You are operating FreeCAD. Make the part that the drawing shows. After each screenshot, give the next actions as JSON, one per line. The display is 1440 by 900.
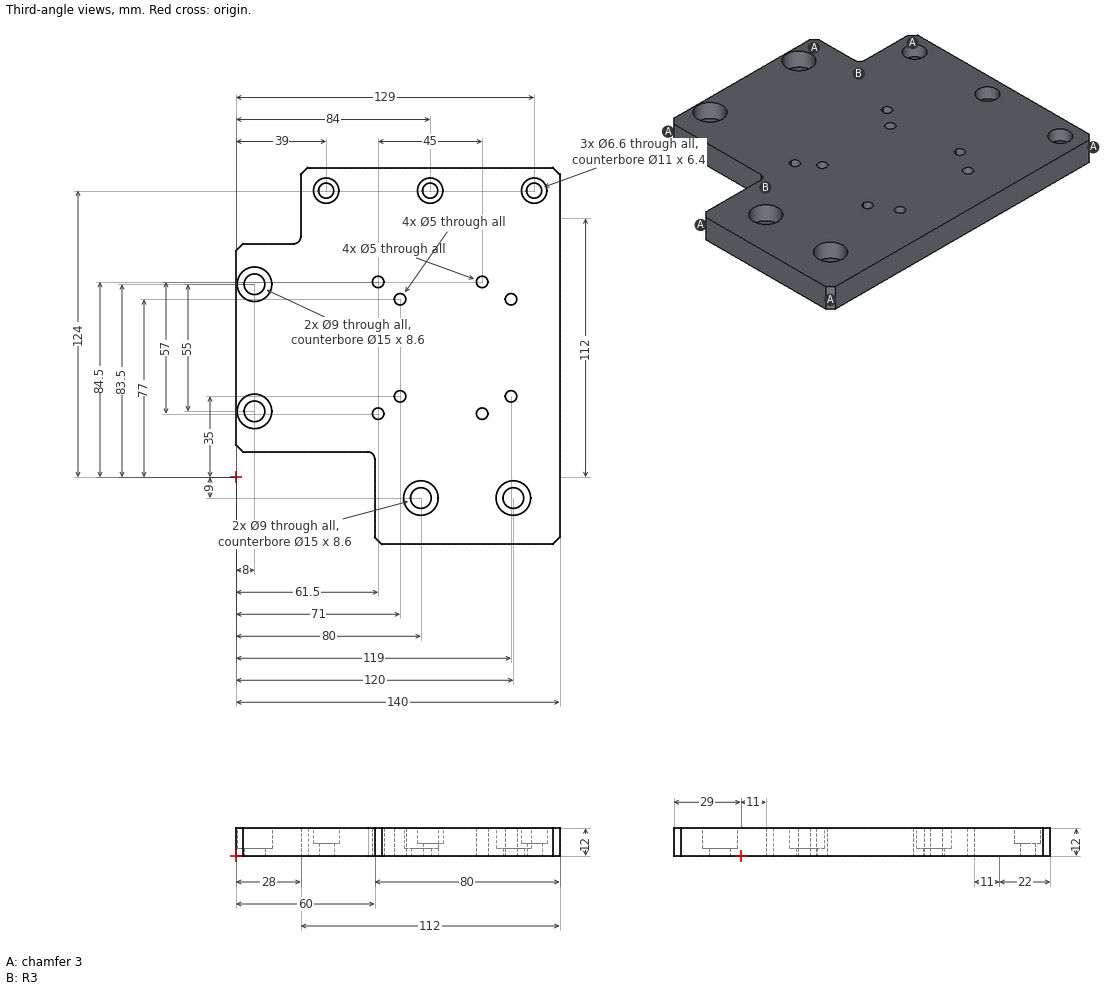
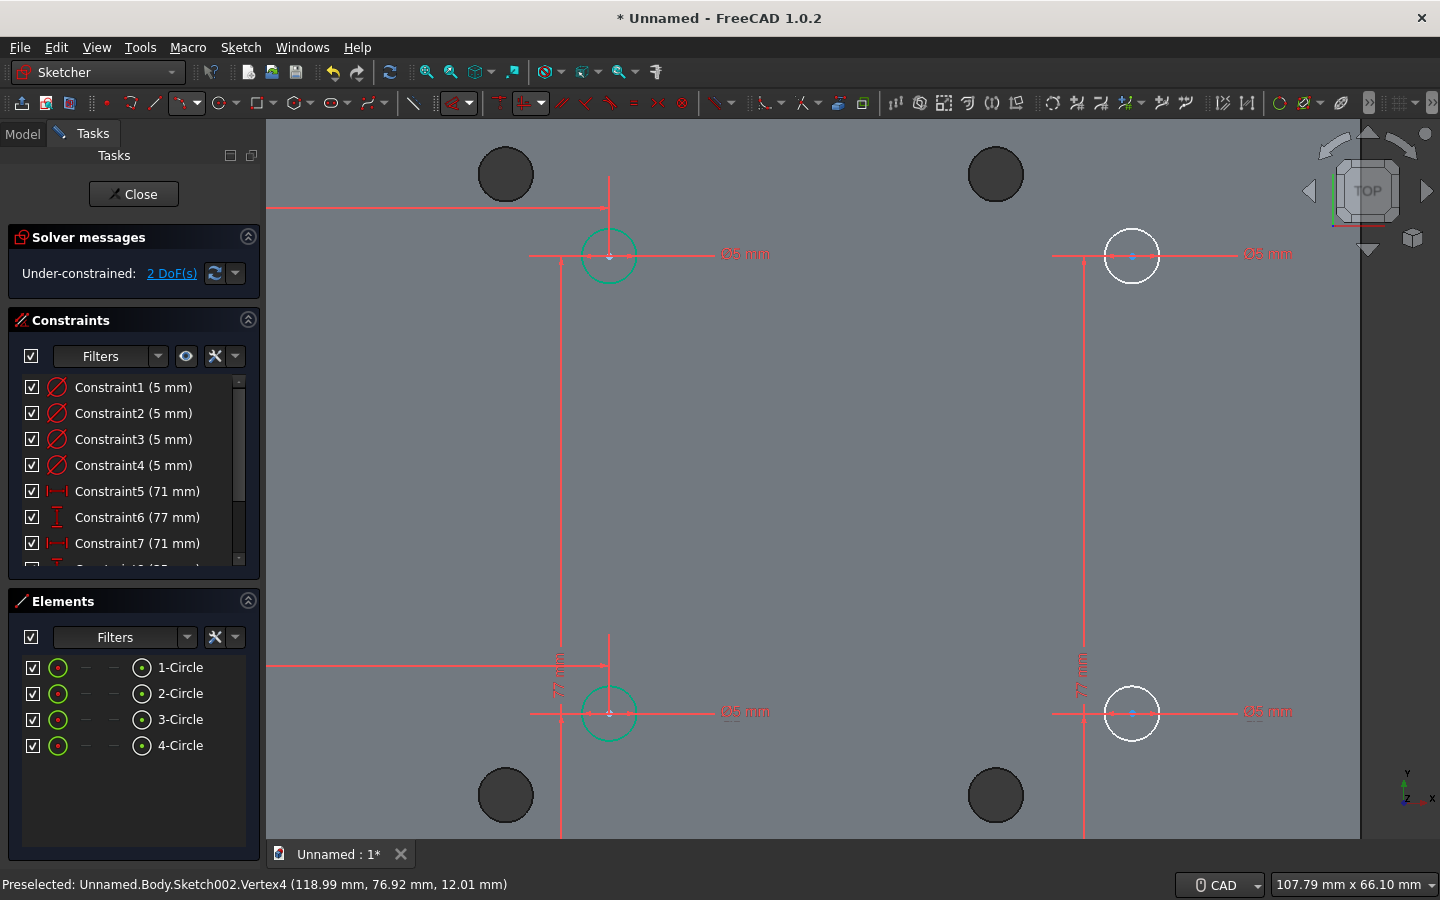
{"action": "left_click", "coordinate": [1132, 714]}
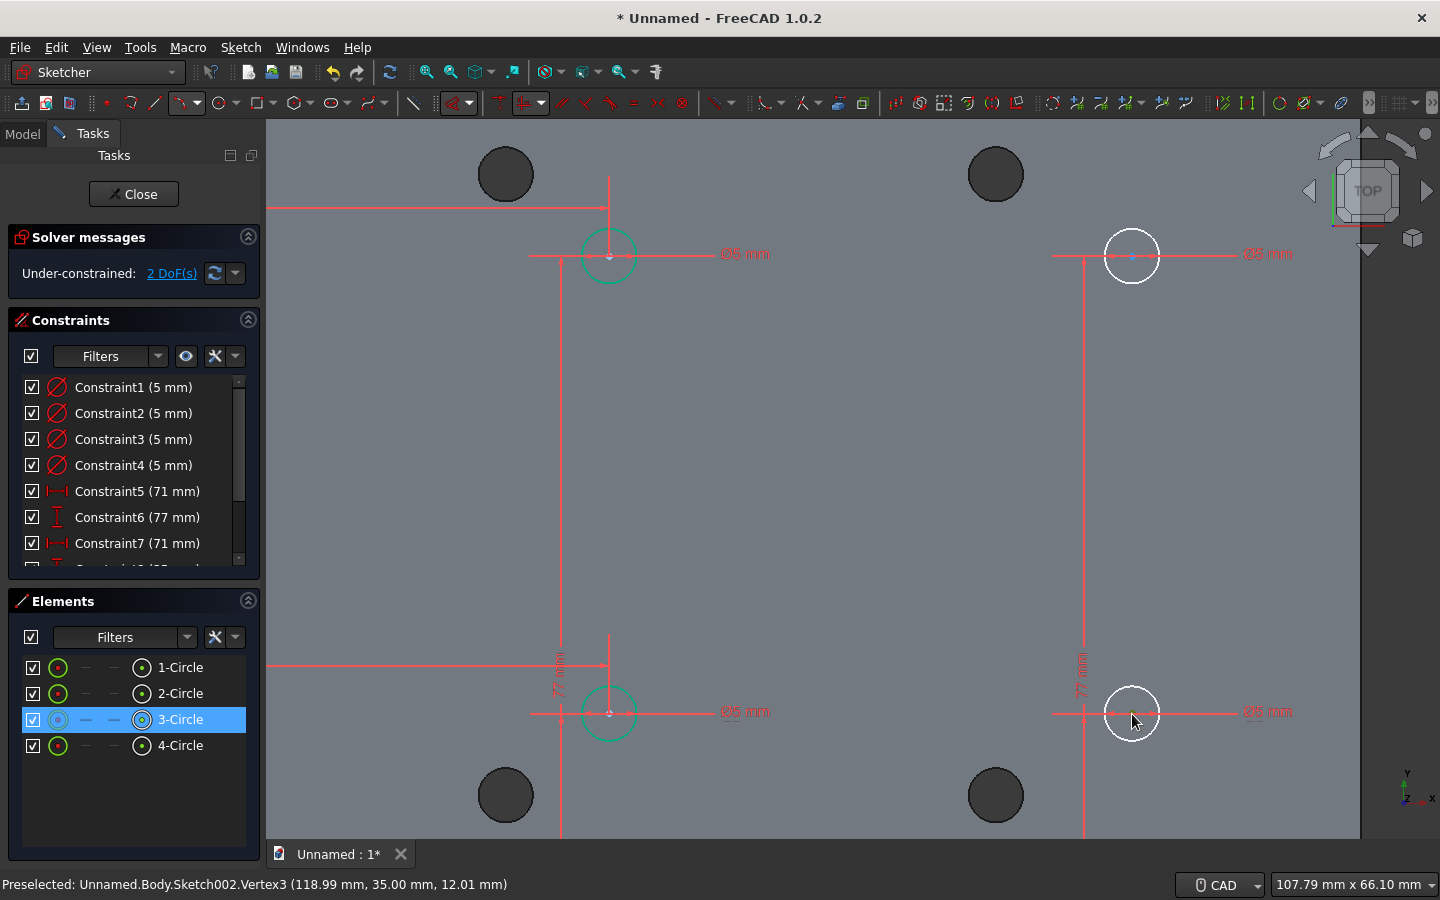
{"action": "key", "text": "l"}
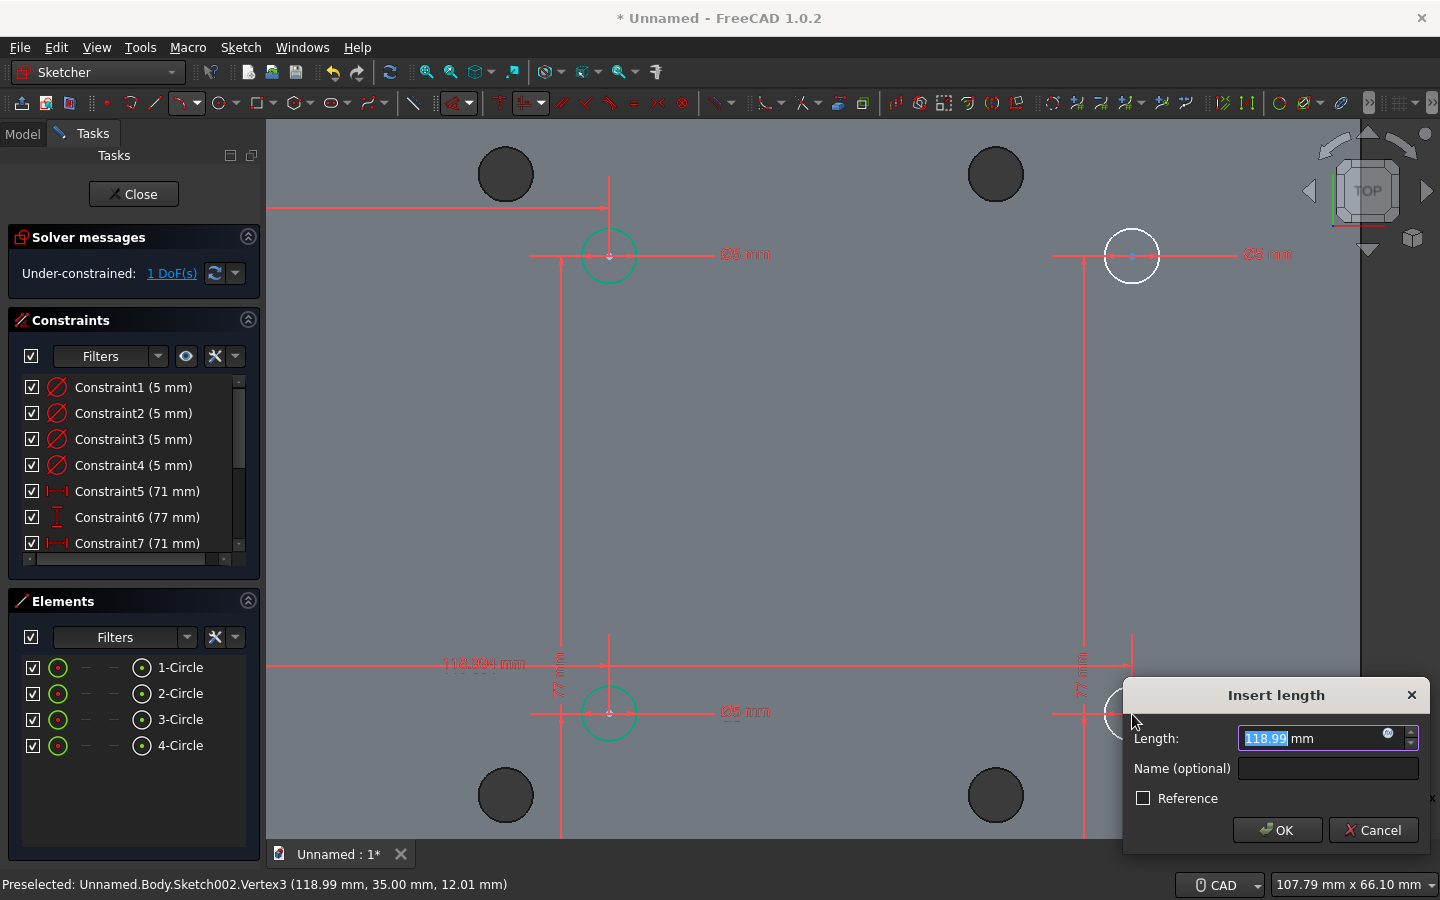
{"action": "type", "text": "119"}
{"action": "key", "text": "Return"}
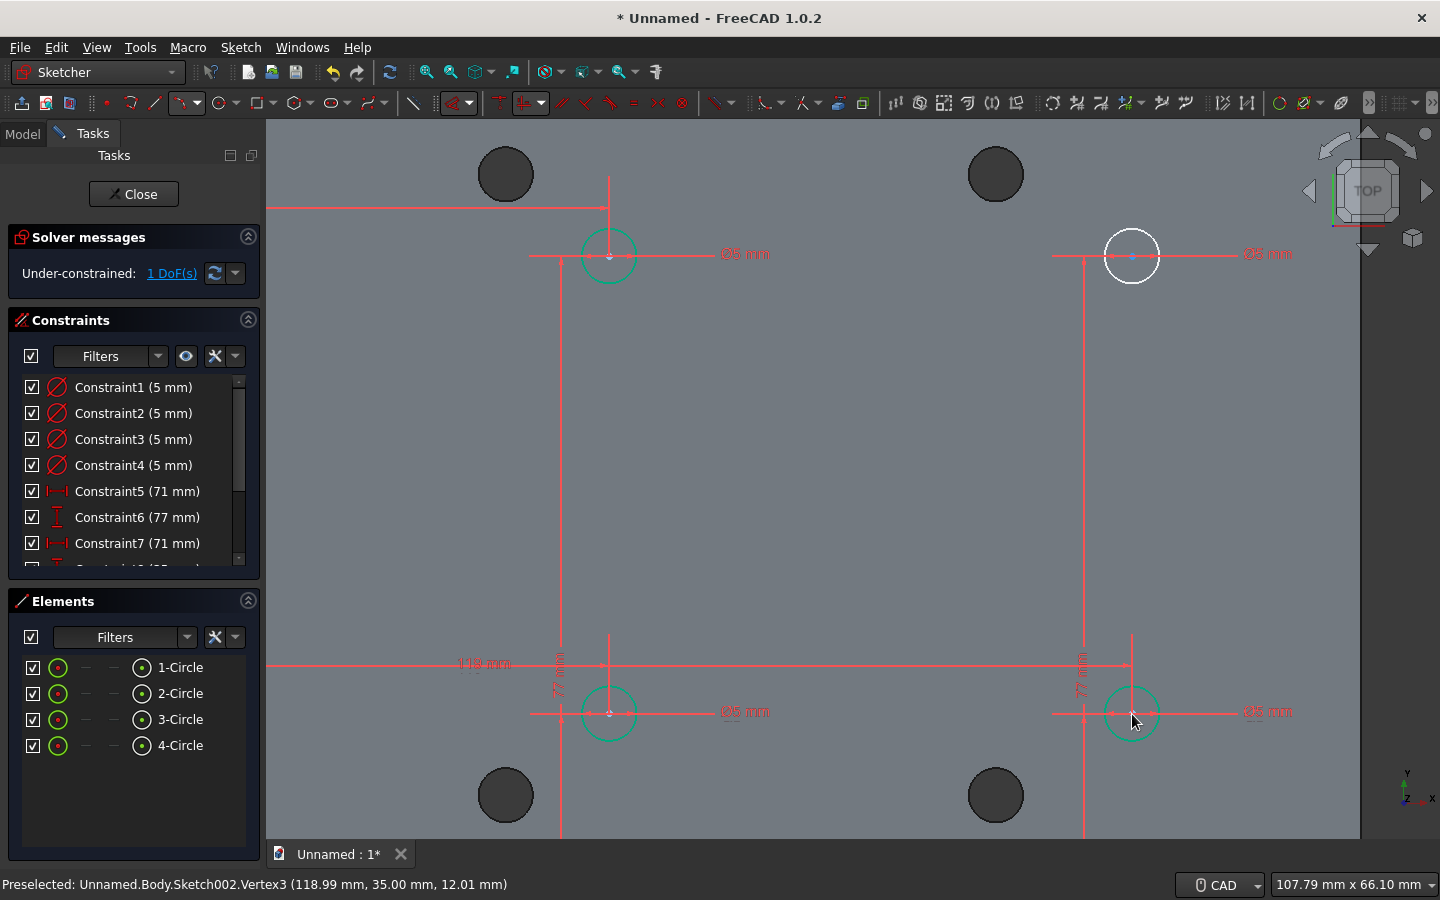
{"action": "left_click", "coordinate": [1132, 256]}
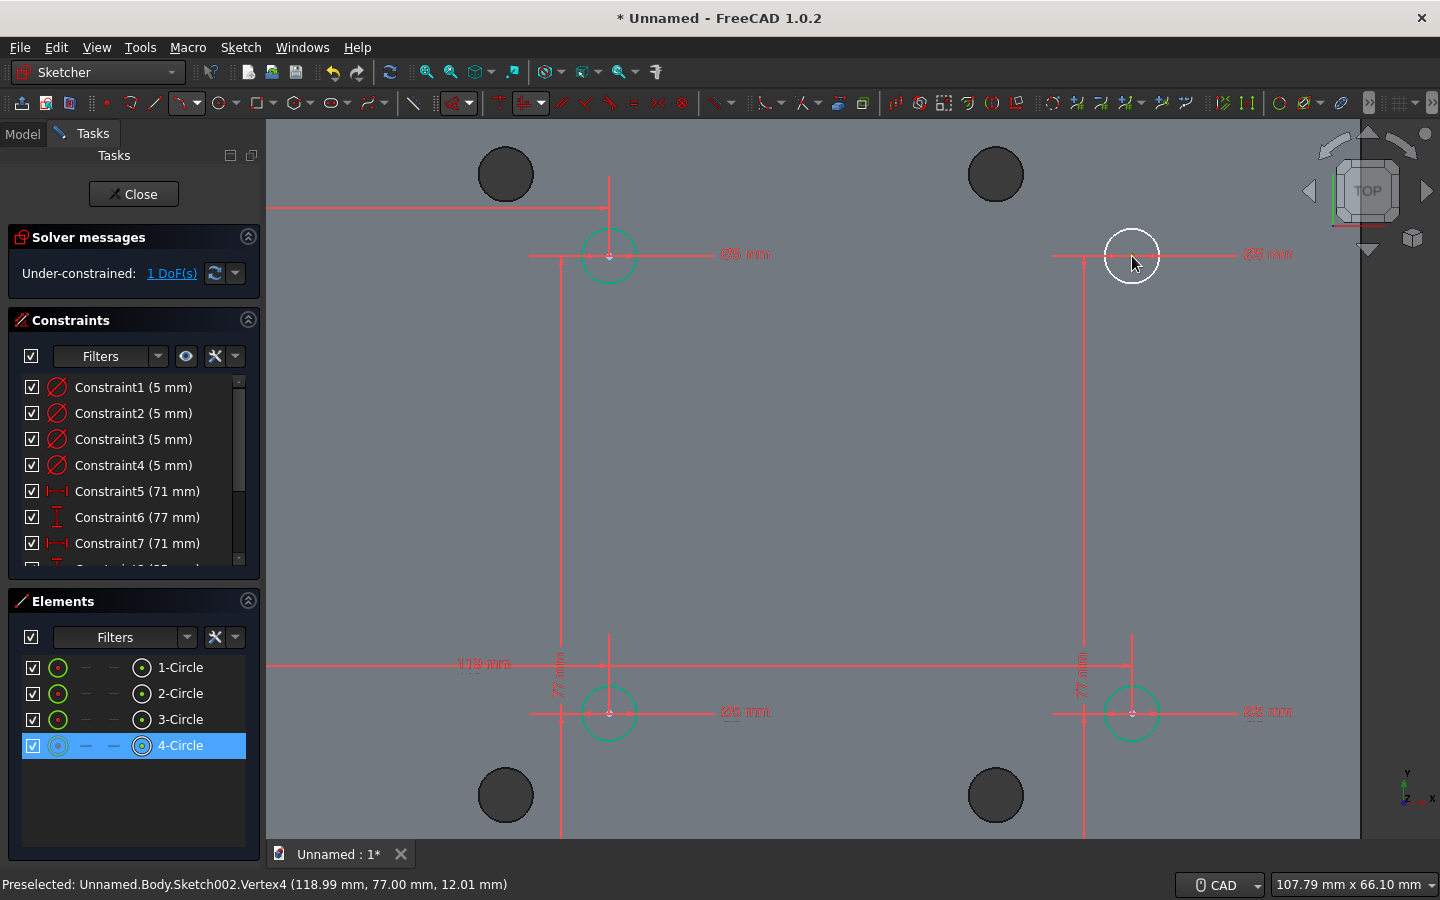
{"action": "left_click", "coordinate": [472, 104]}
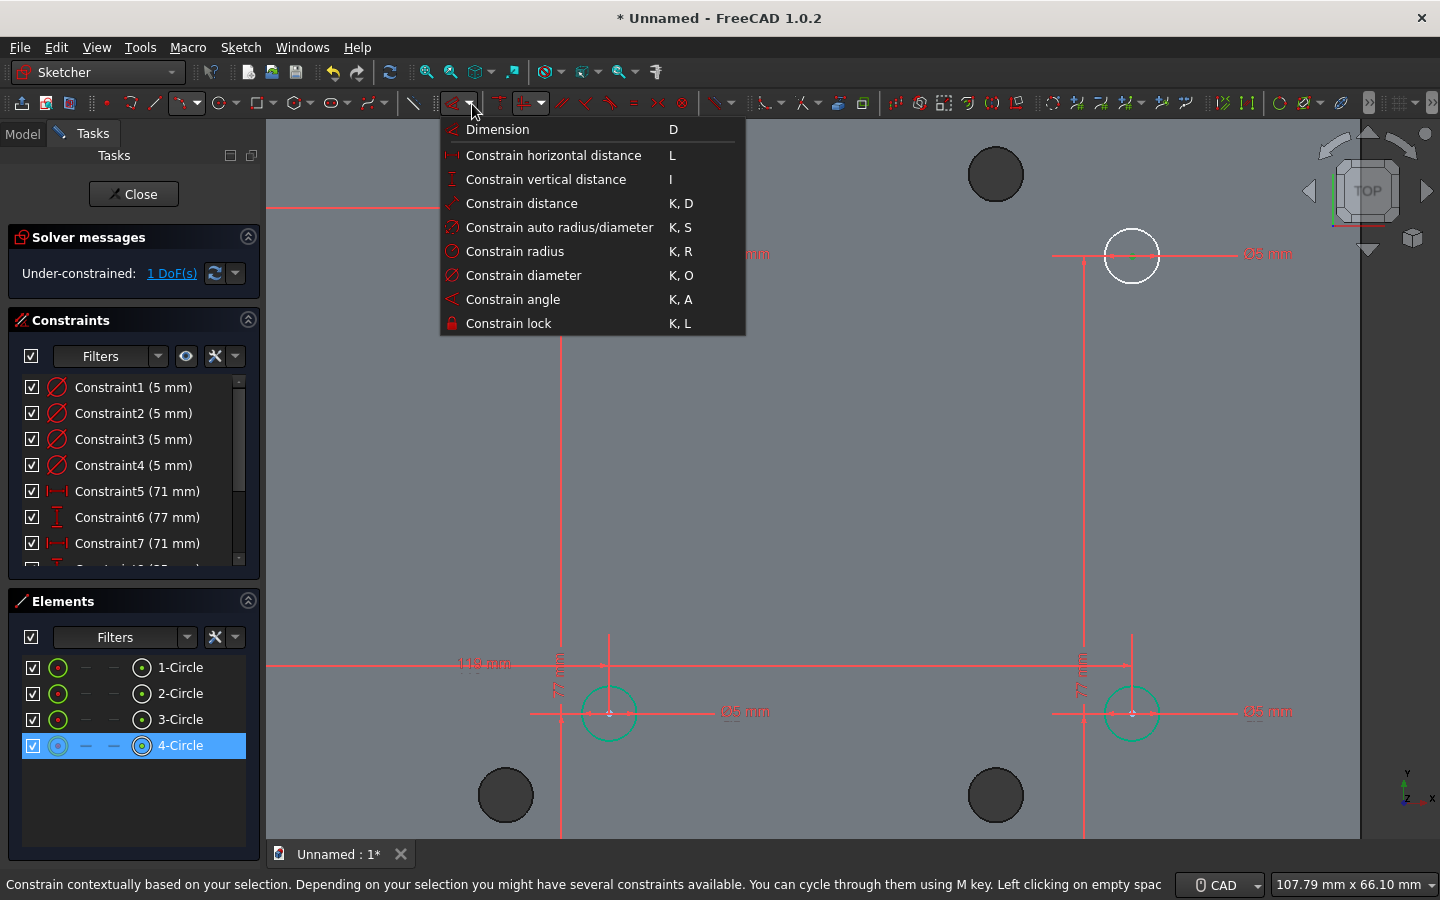
{"action": "left_click", "coordinate": [593, 155]}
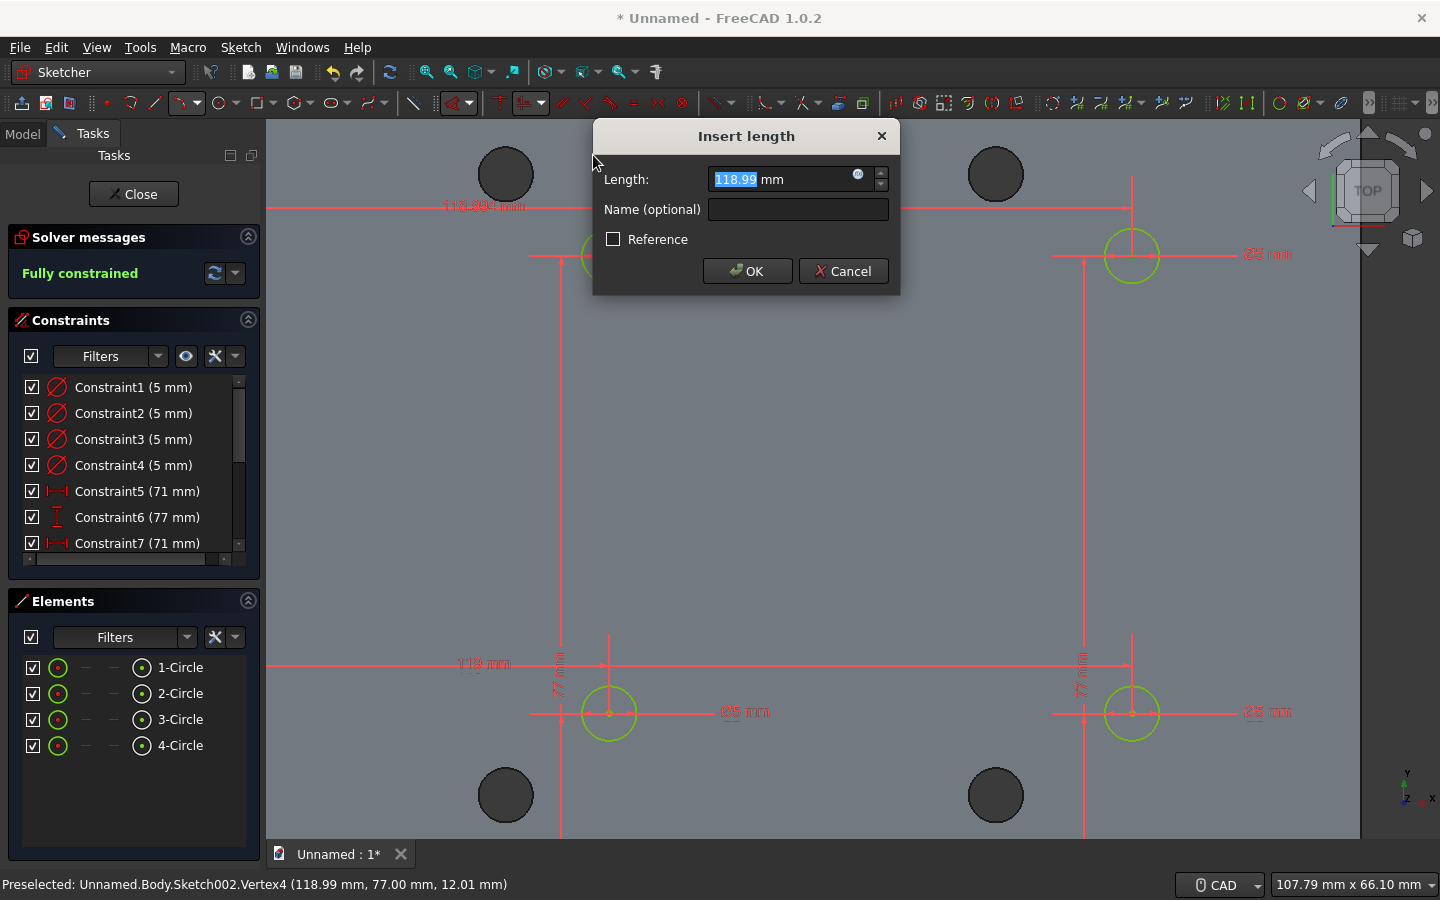
{"action": "type", "text": "119"}
{"action": "key", "text": "Return"}